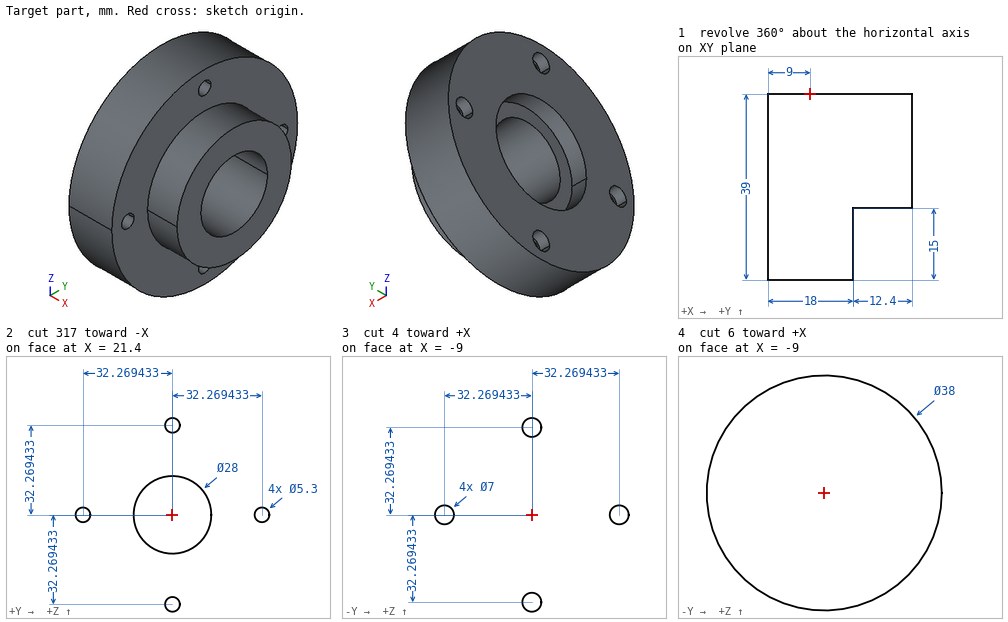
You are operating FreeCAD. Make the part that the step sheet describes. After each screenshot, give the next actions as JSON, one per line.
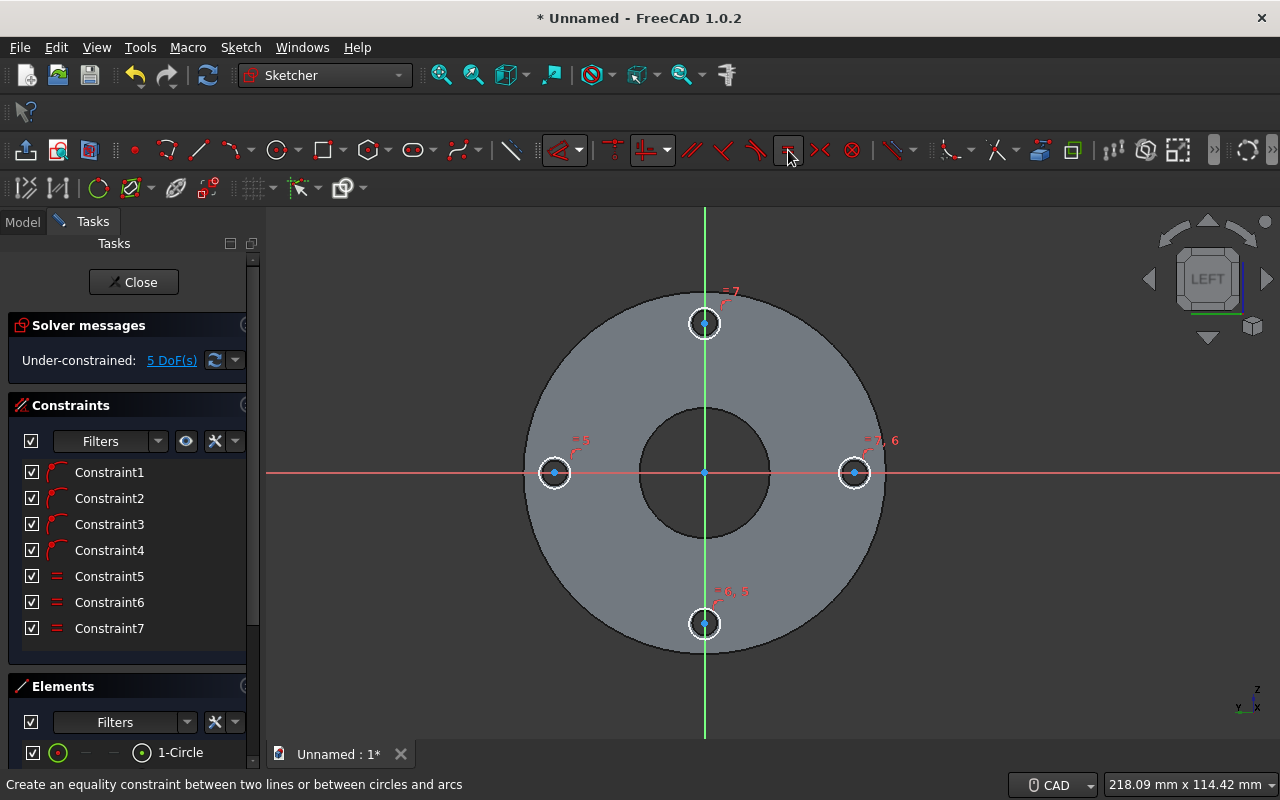
{"action": "scroll", "coordinate": [566, 462], "scroll_direction": "up", "scroll_amount": 2}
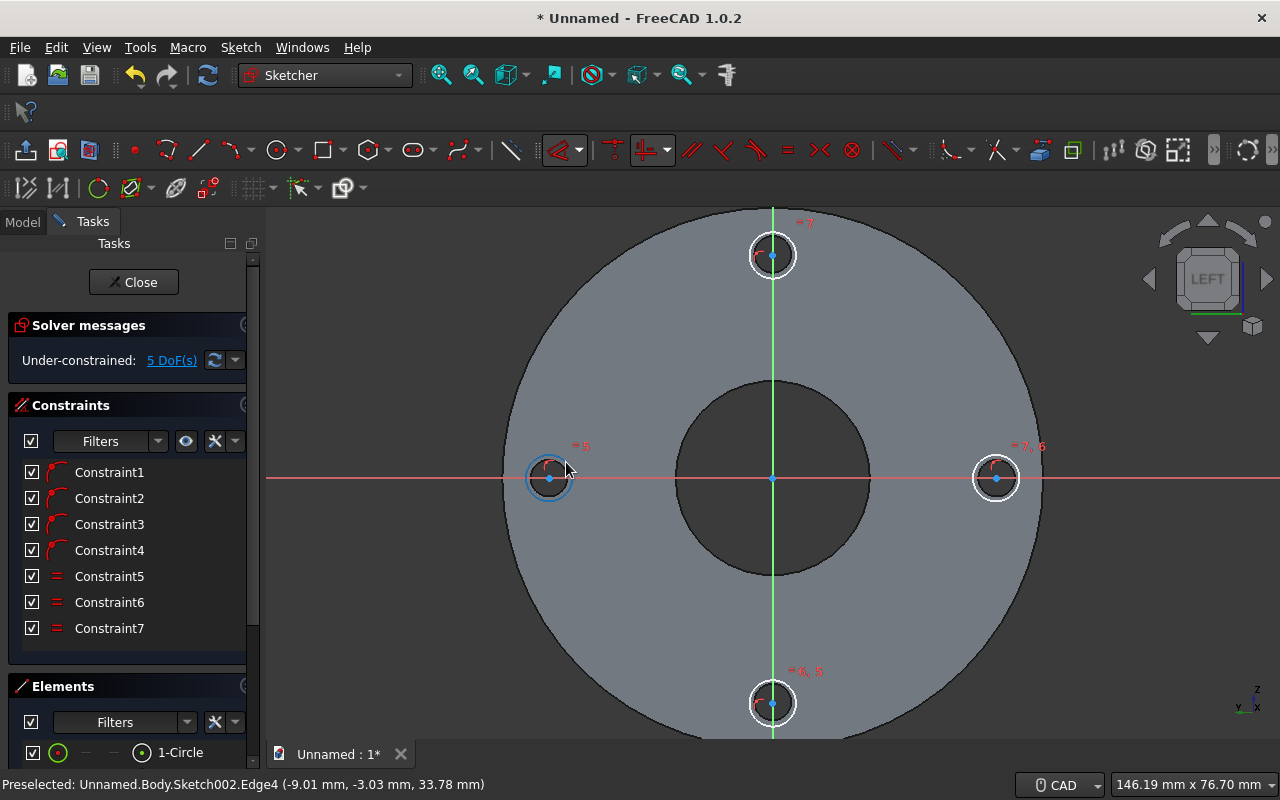
{"action": "left_click", "coordinate": [565, 462]}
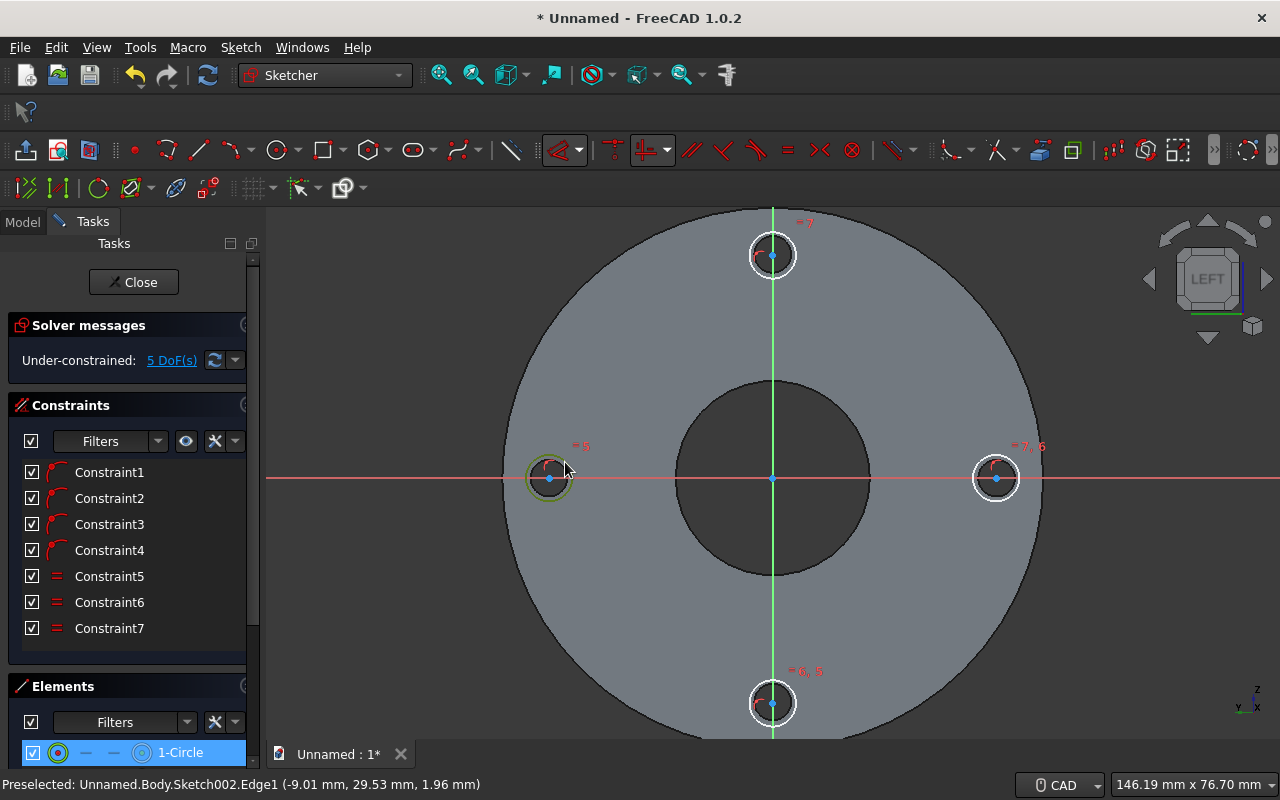
{"action": "key", "text": "k o"}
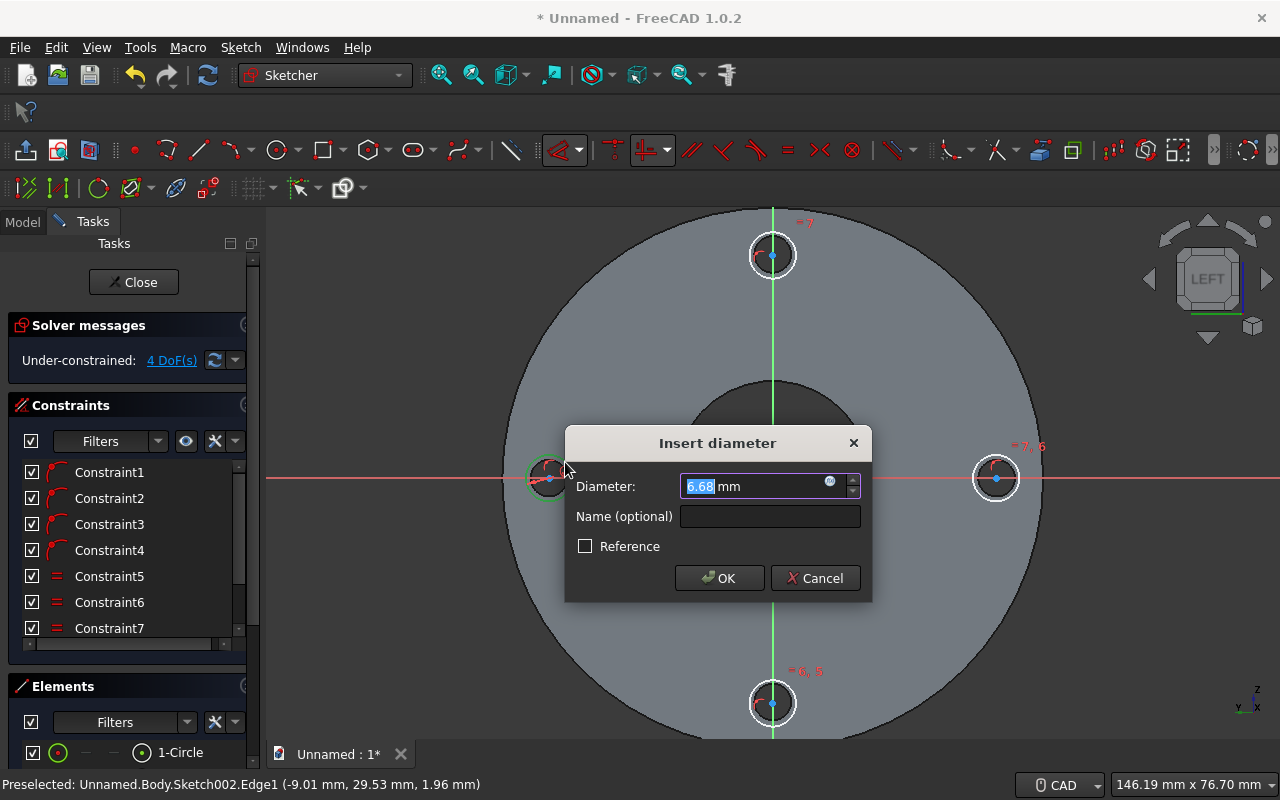
{"action": "type", "text": "7"}
{"action": "key", "text": "Return"}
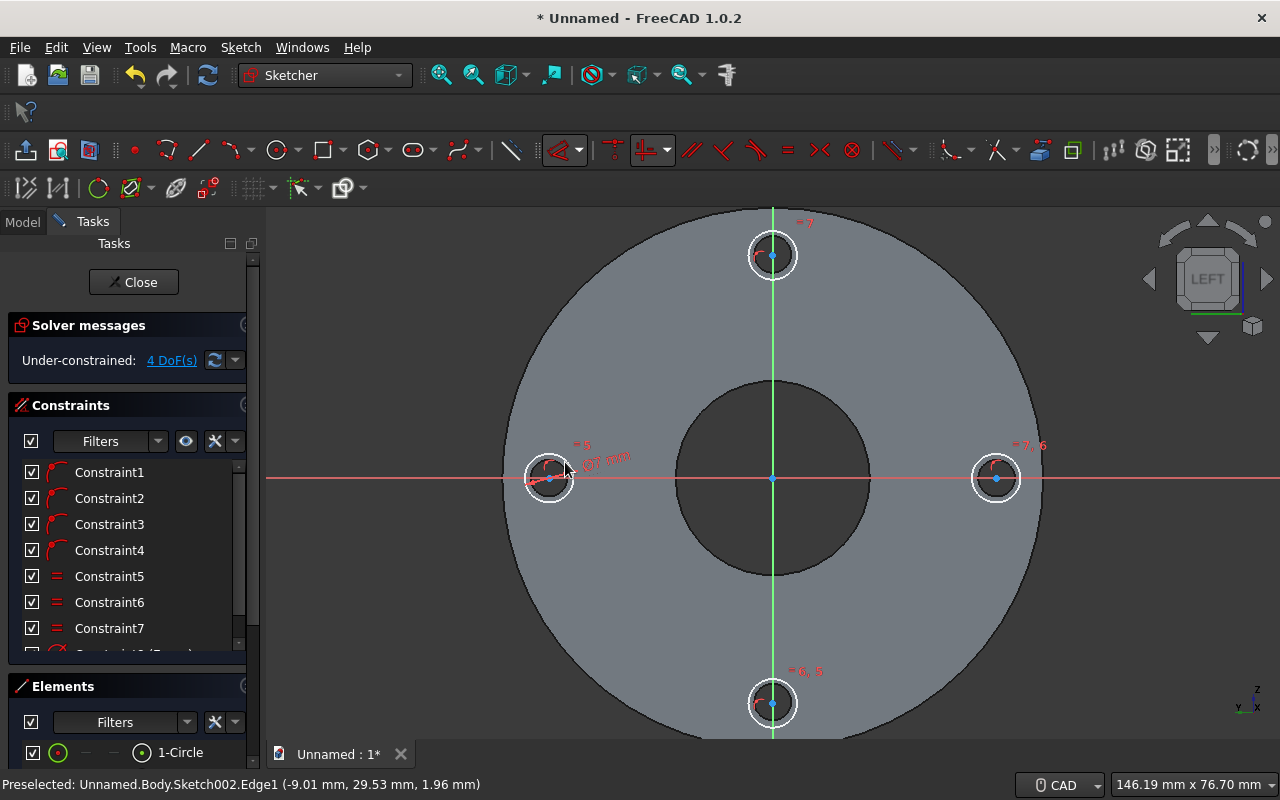
{"action": "left_click", "coordinate": [549, 478]}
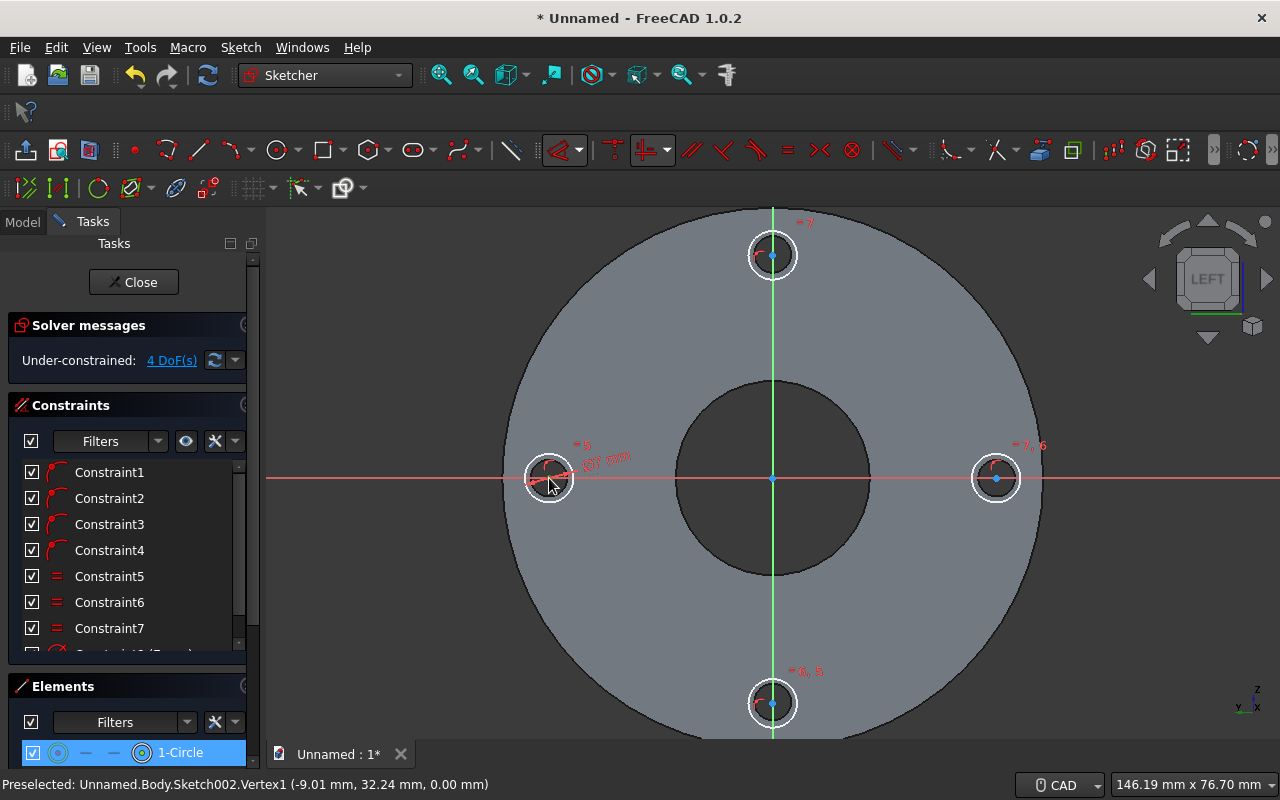
{"action": "left_click", "coordinate": [582, 150]}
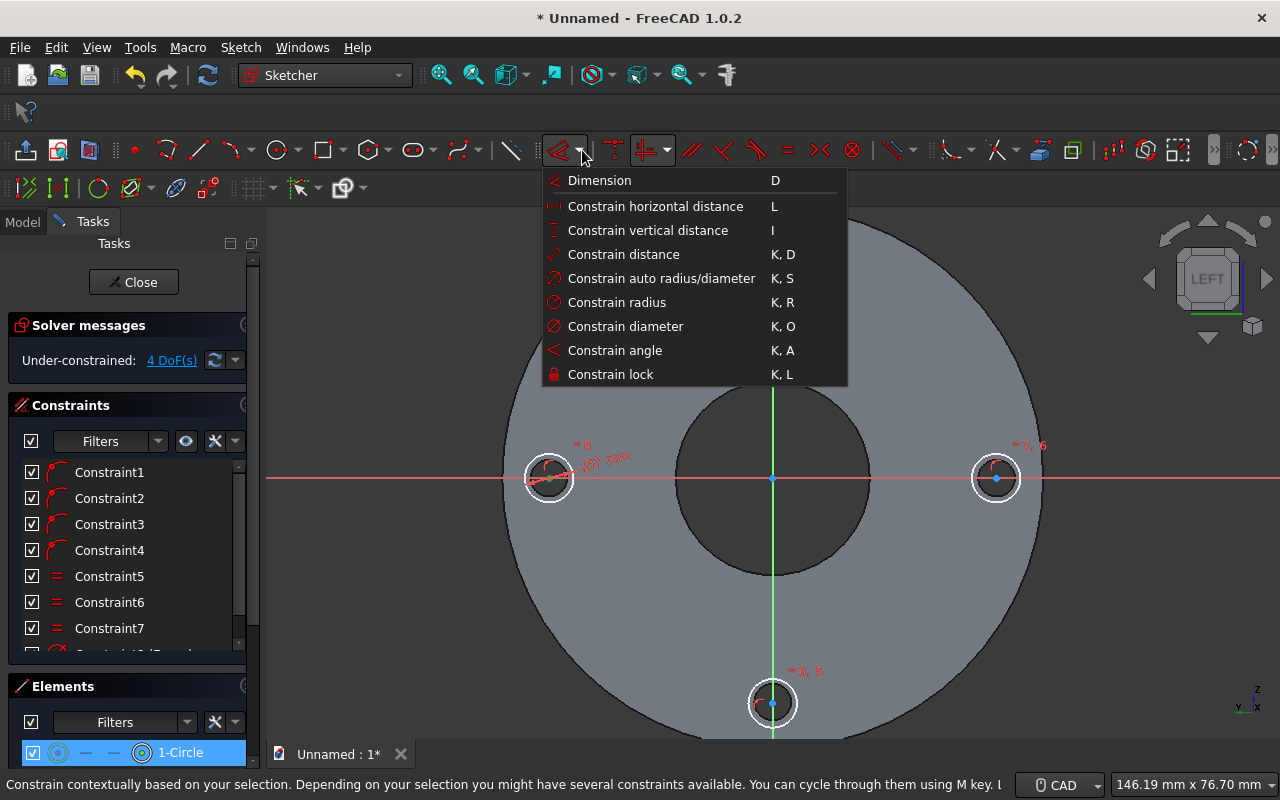
{"action": "left_click", "coordinate": [695, 206]}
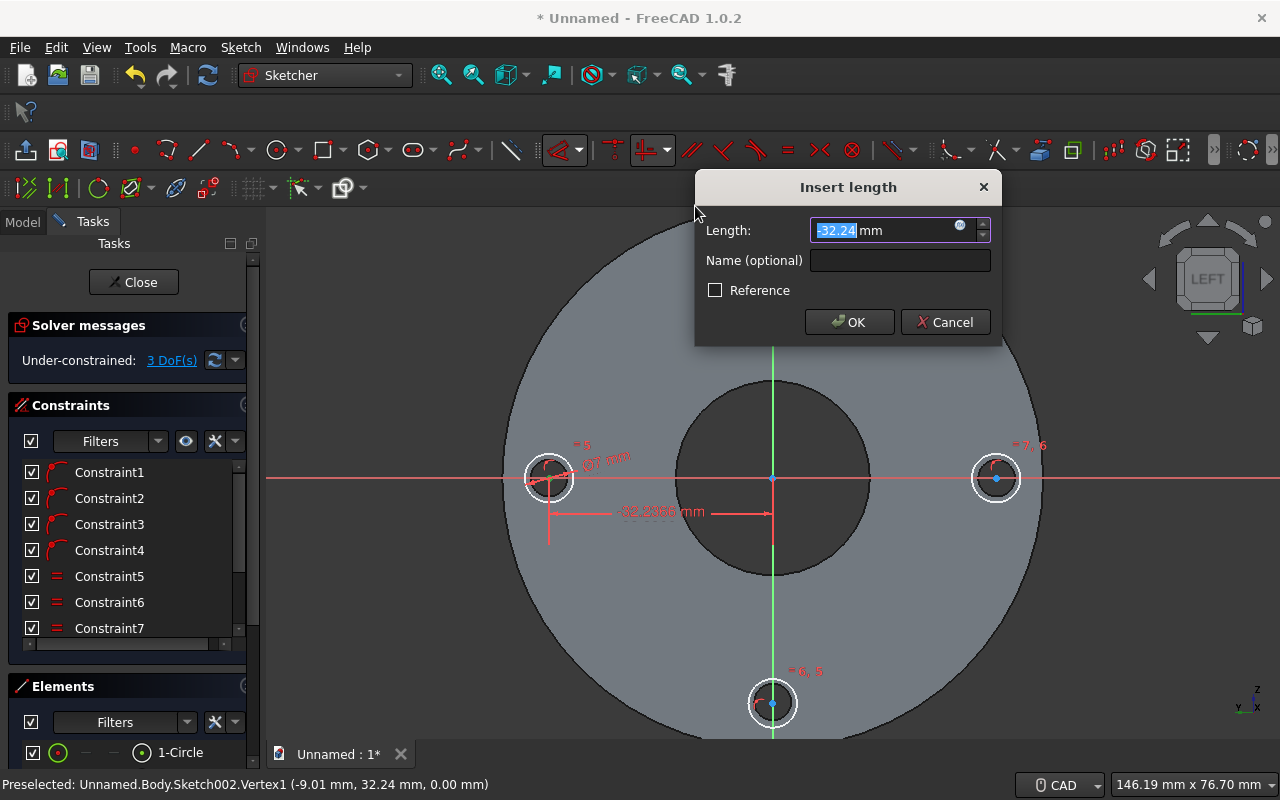
{"action": "type", "text": "-32.269433"}
{"action": "key", "text": "Return"}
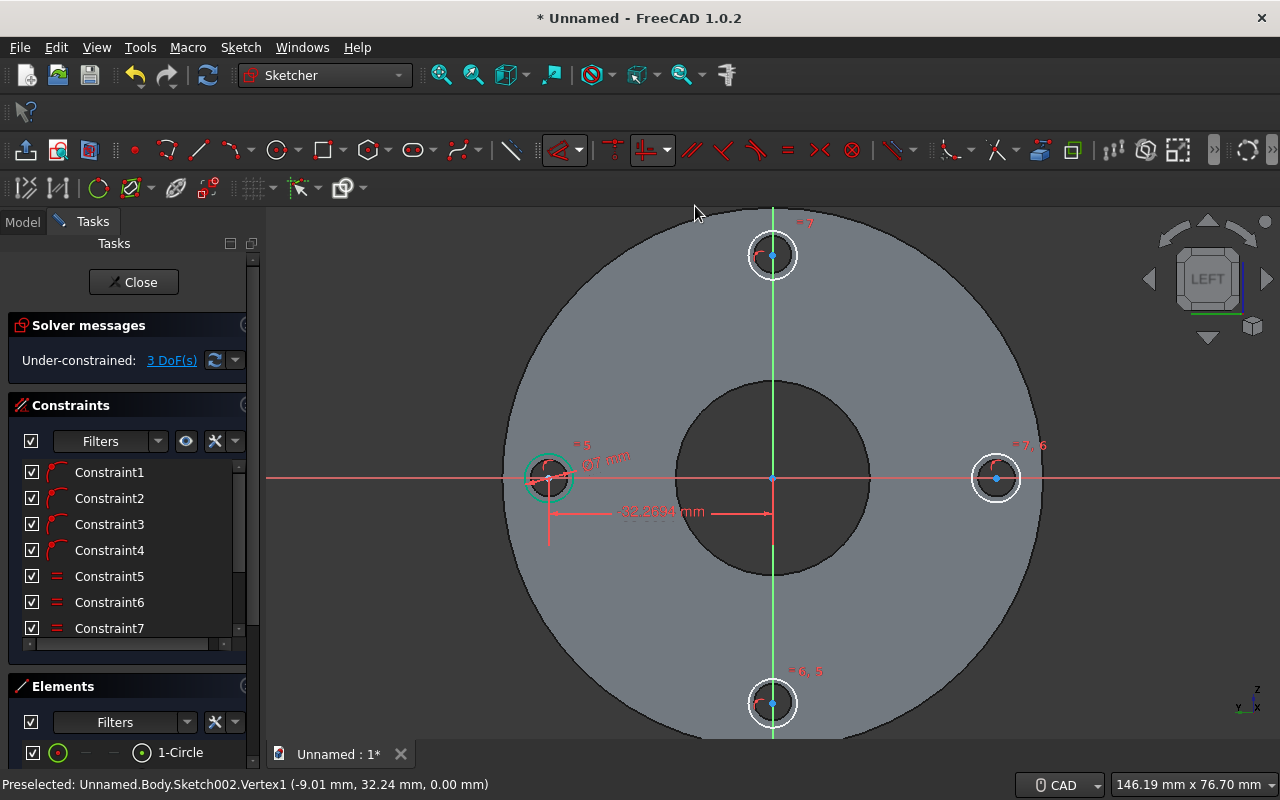
{"action": "left_click", "coordinate": [773, 703]}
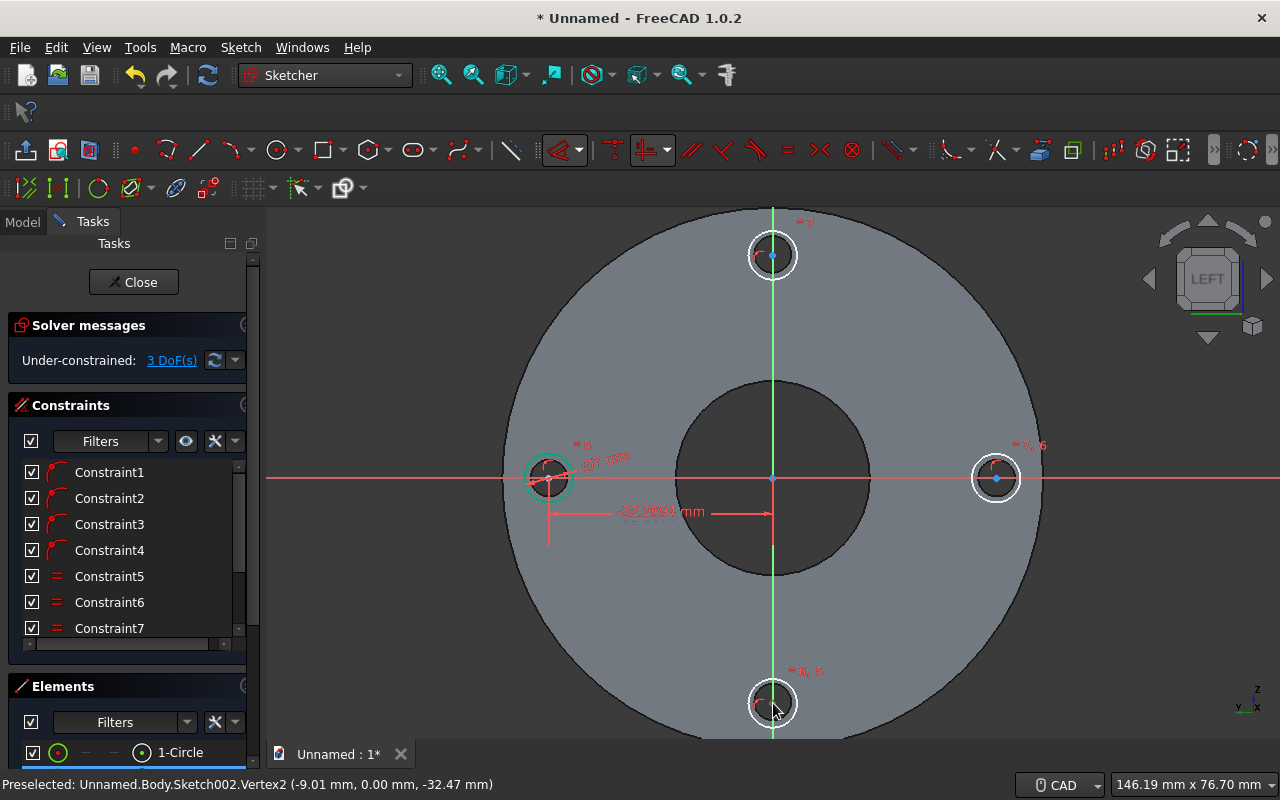
{"action": "left_click", "coordinate": [582, 150]}